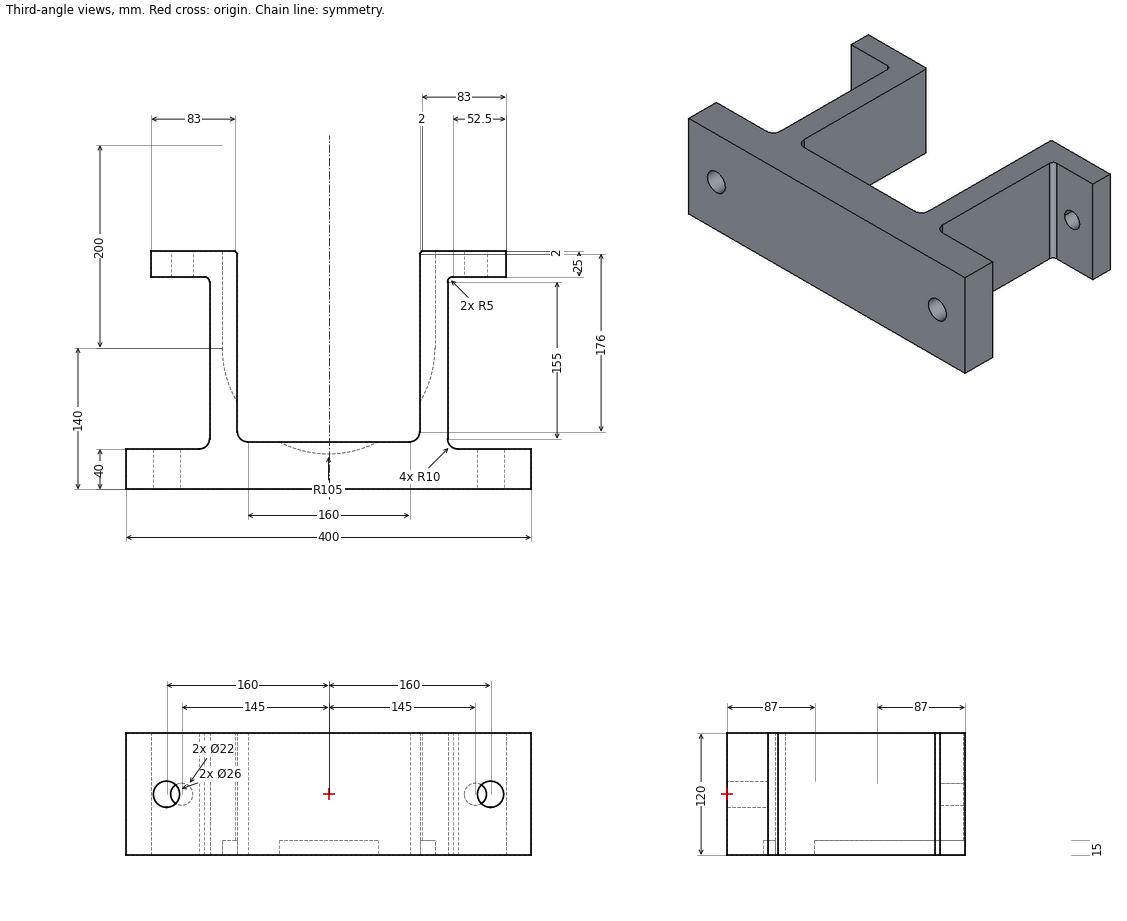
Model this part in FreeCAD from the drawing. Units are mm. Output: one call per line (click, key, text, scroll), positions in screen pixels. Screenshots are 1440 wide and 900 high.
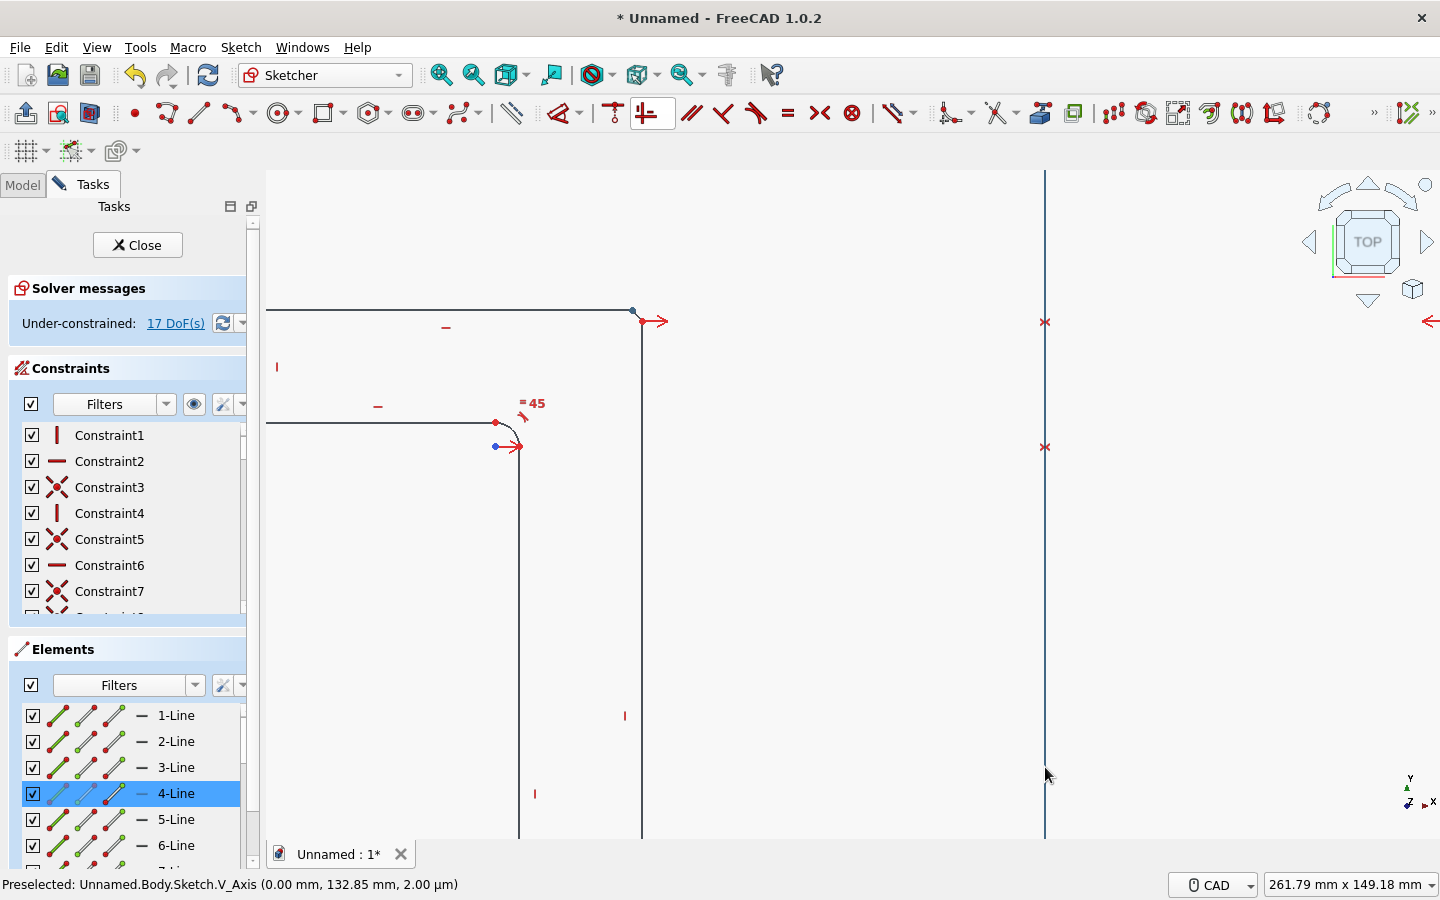
click(820, 114)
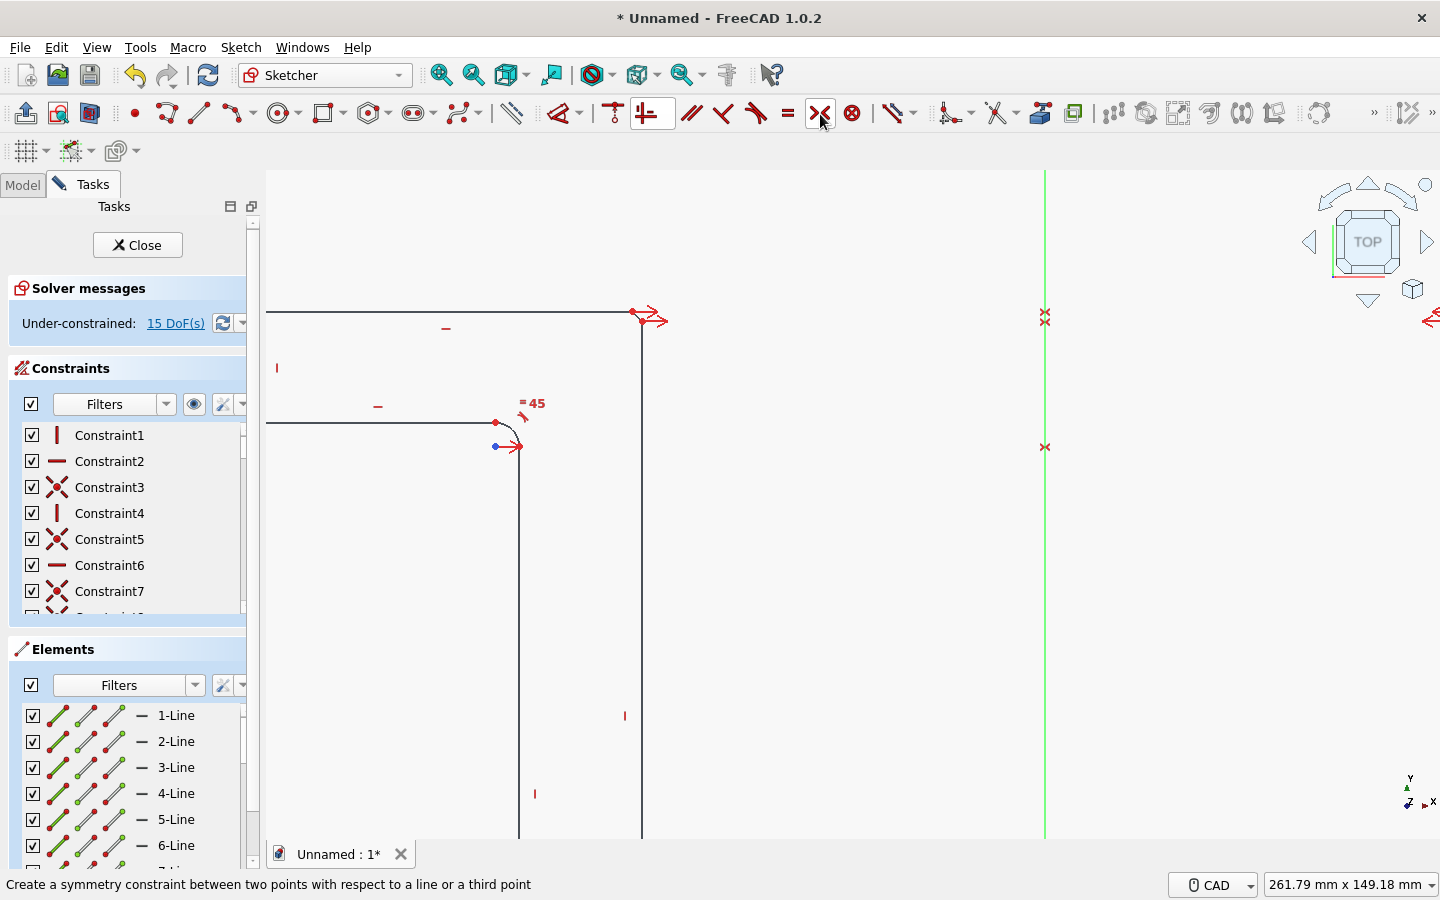
scroll(633, 311, down, 5)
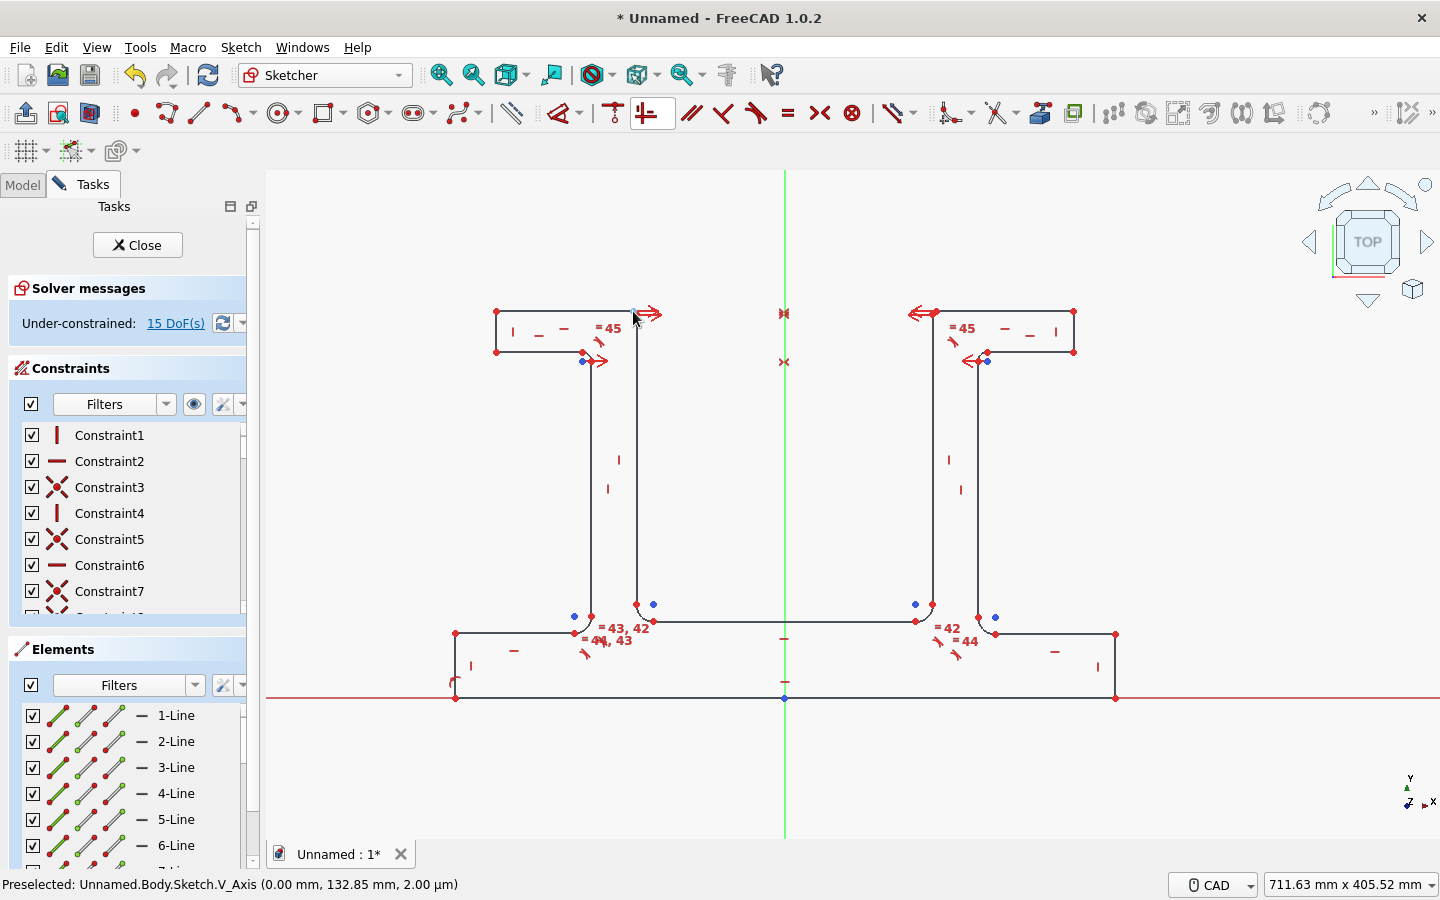
click(455, 633)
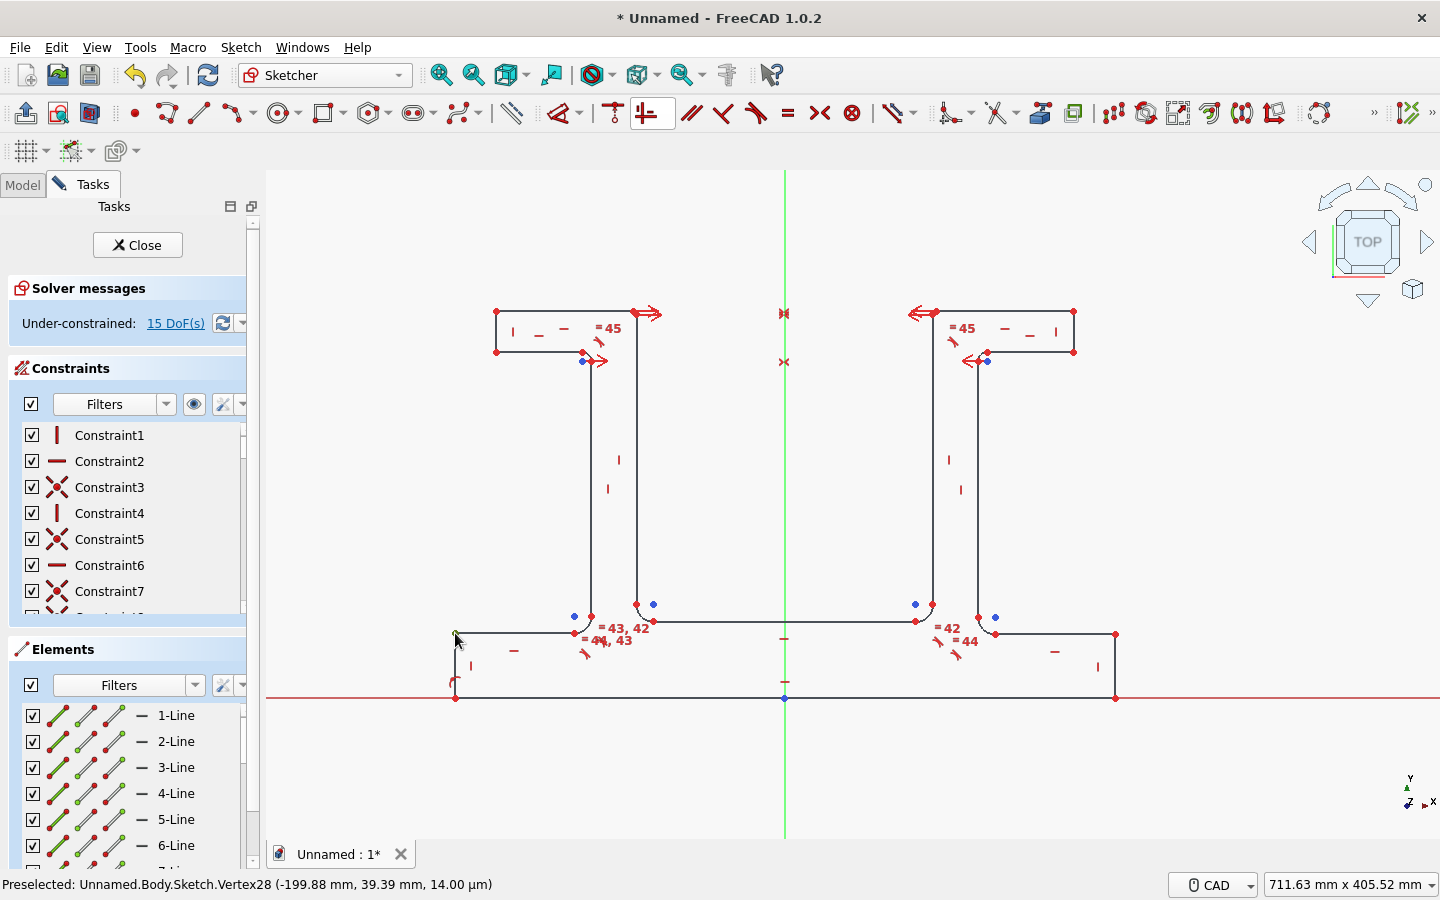
click(1115, 634)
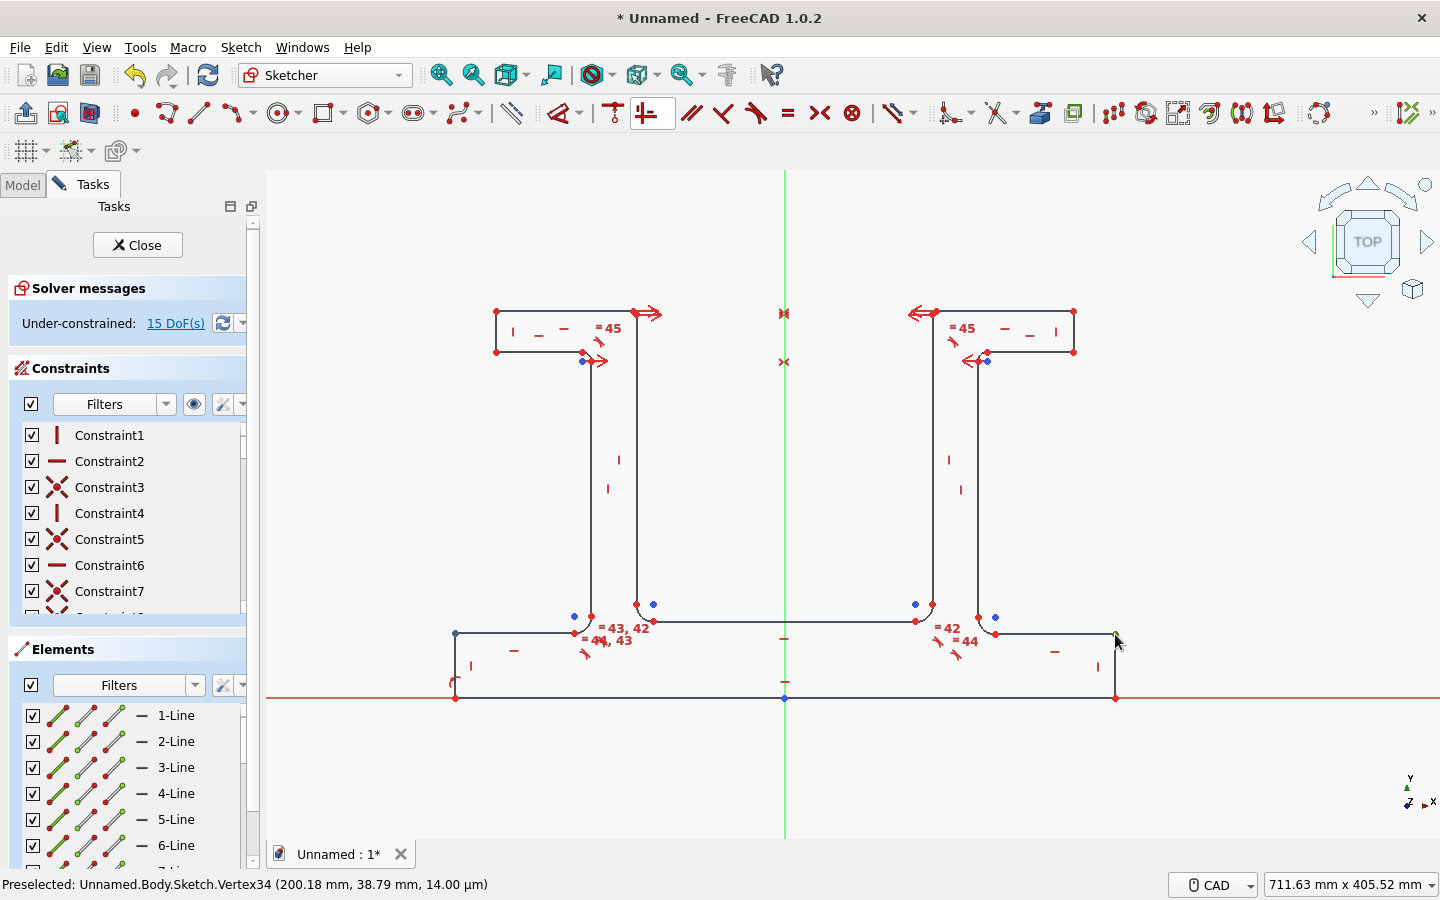
click(785, 767)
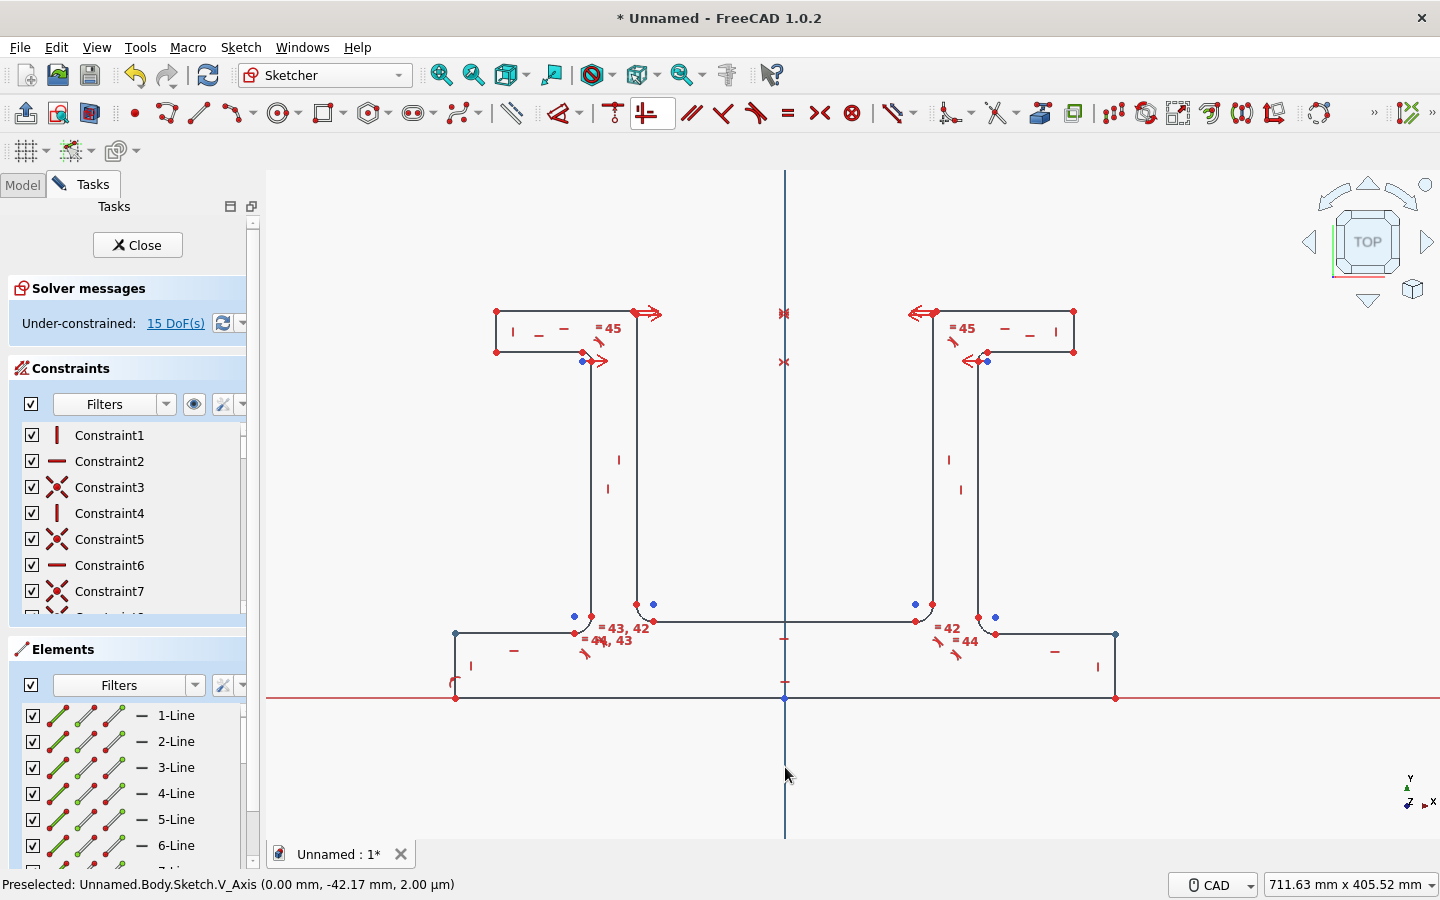
click(820, 114)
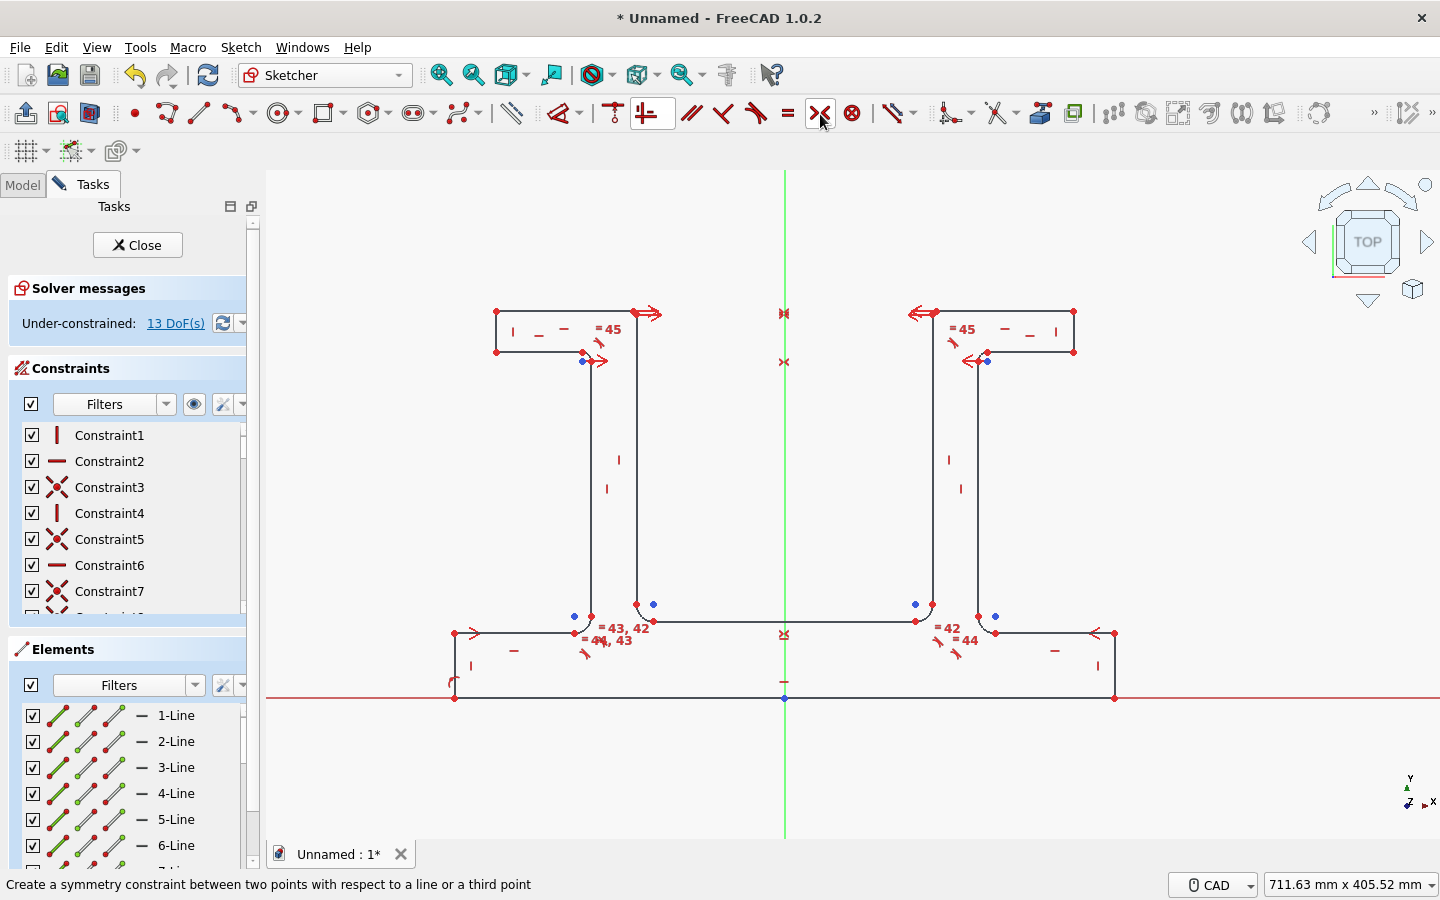
click(558, 114)